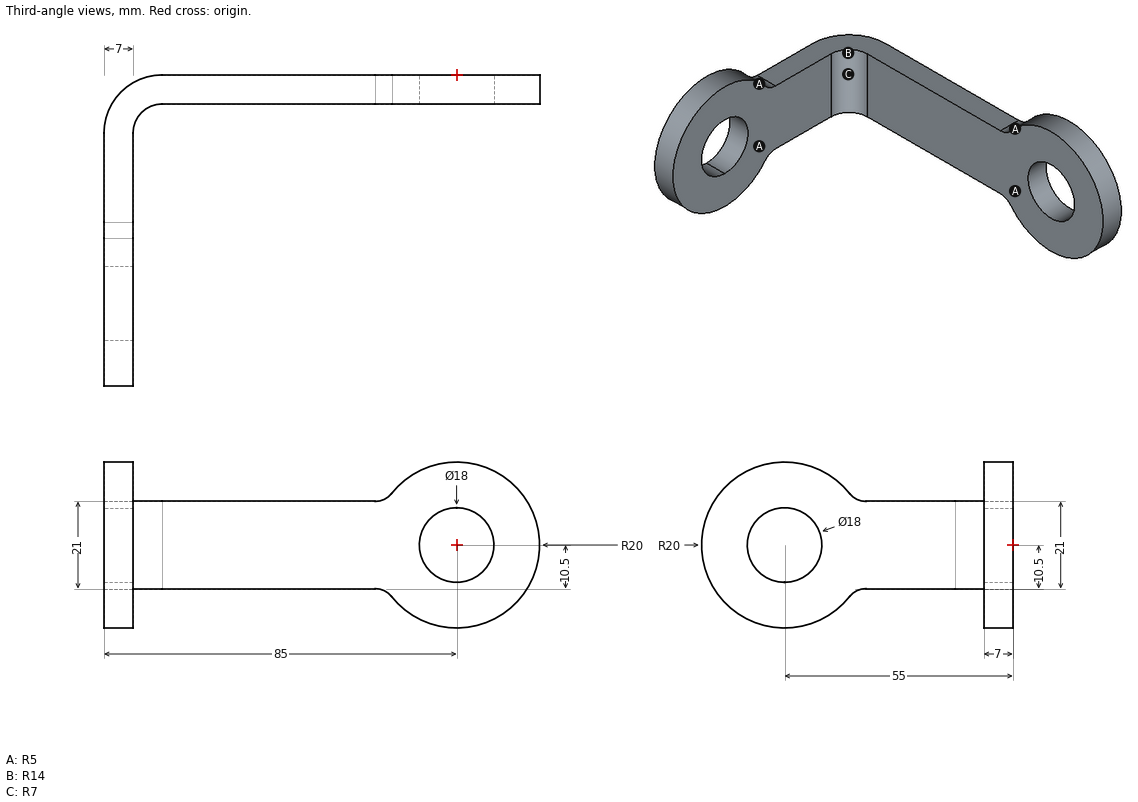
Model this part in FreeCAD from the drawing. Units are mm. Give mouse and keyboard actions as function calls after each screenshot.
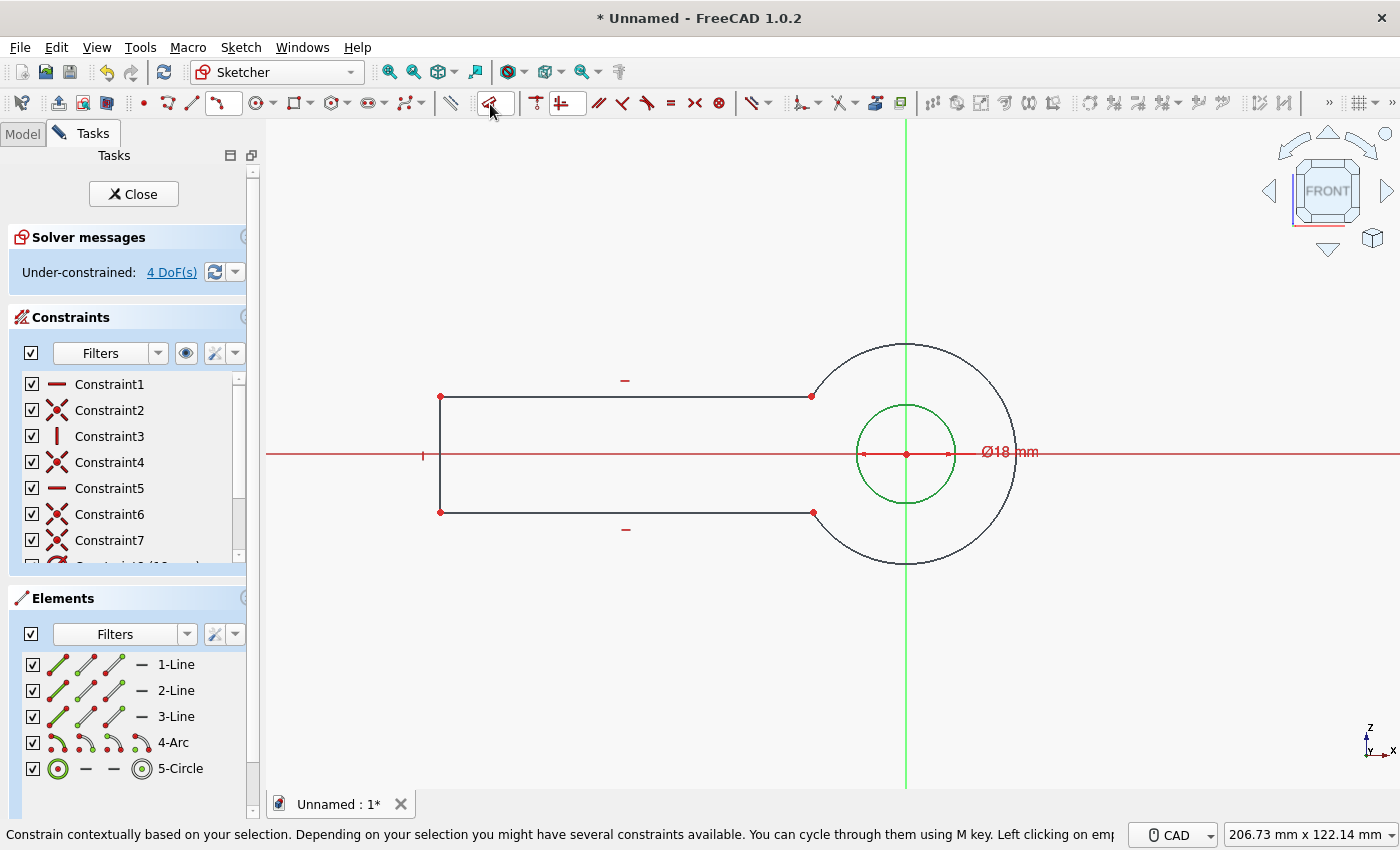
click(963, 548)
click(980, 575)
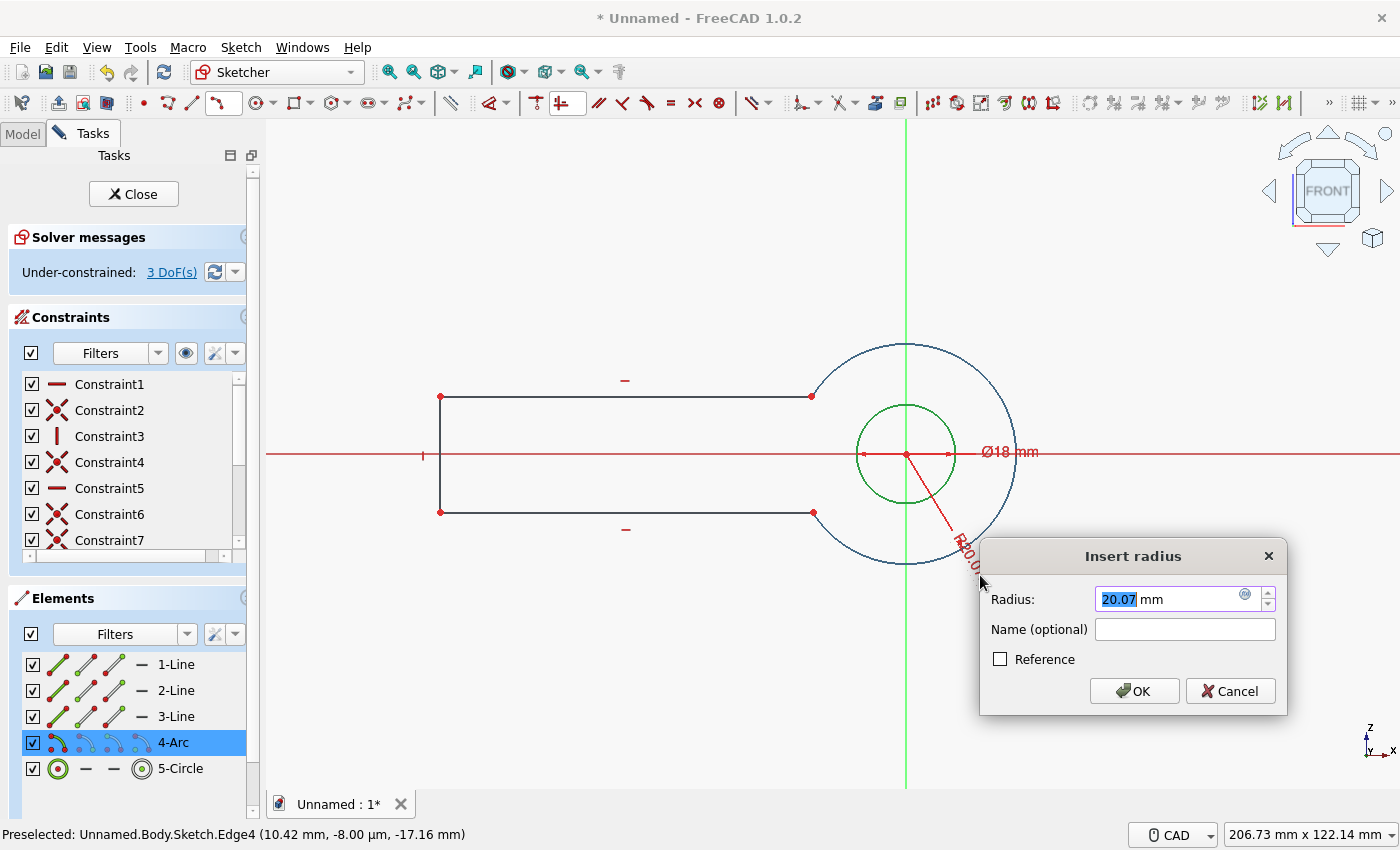
text(20)
key(Return)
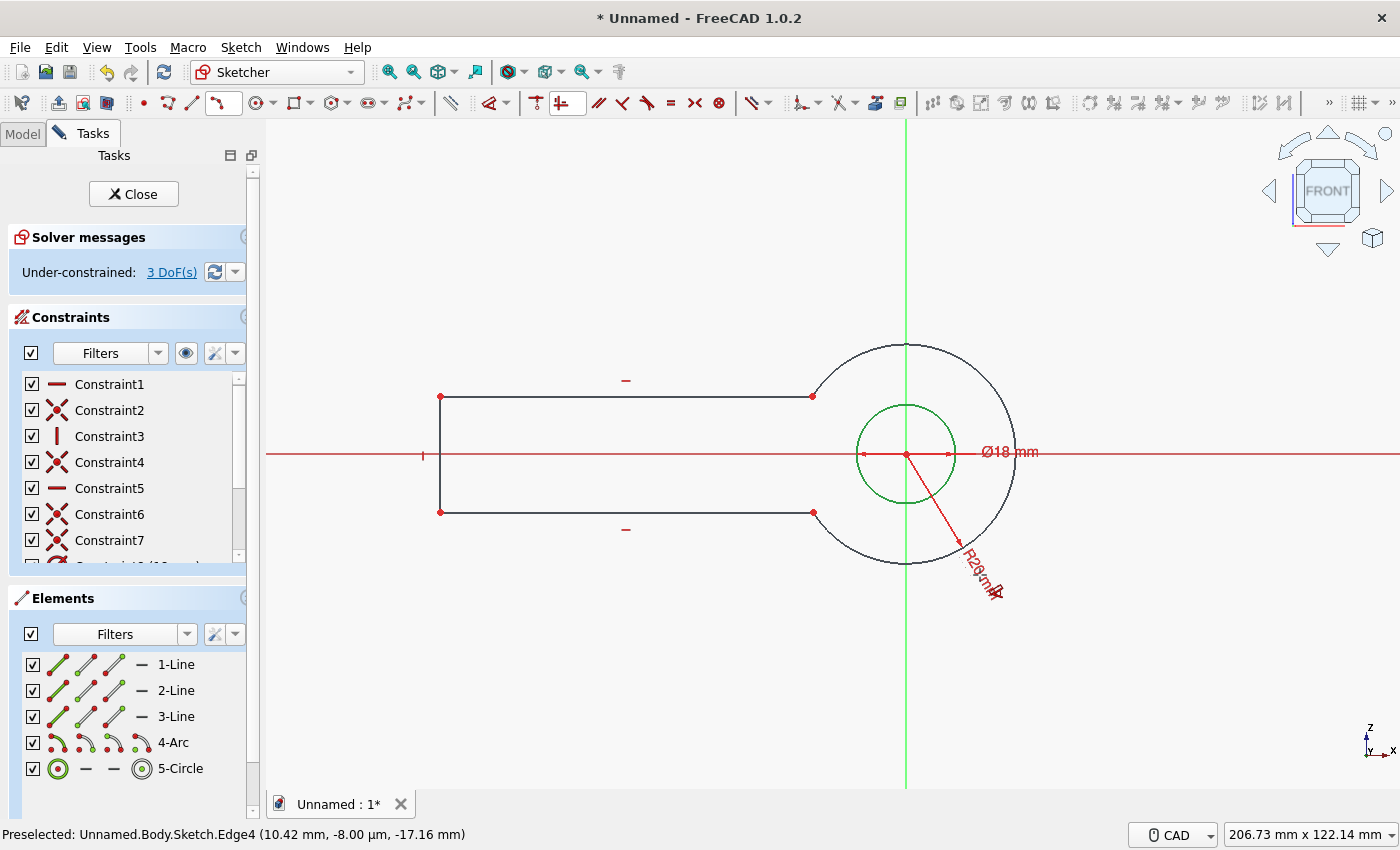
click(440, 478)
click(406, 428)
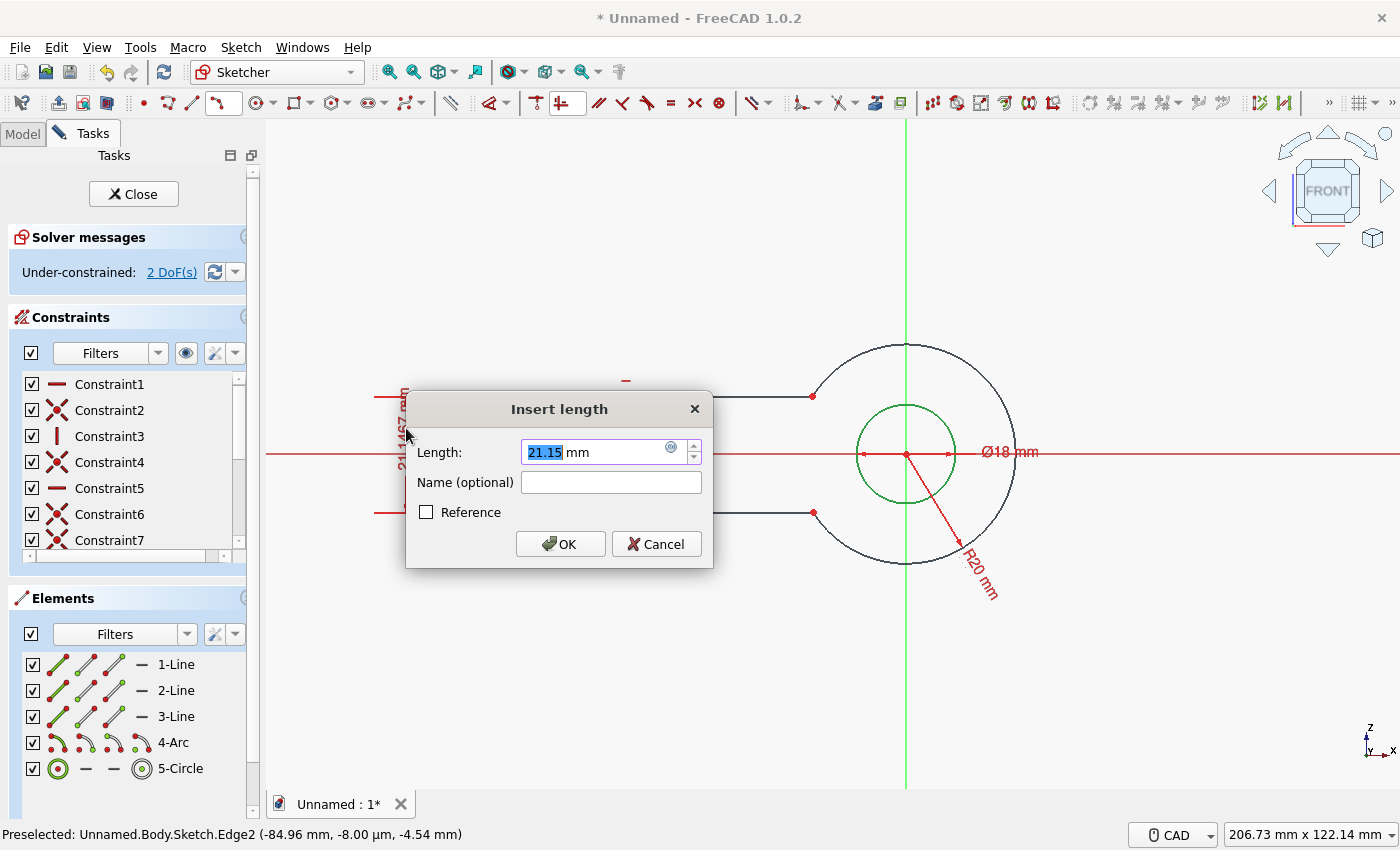
text(21)
key(Return)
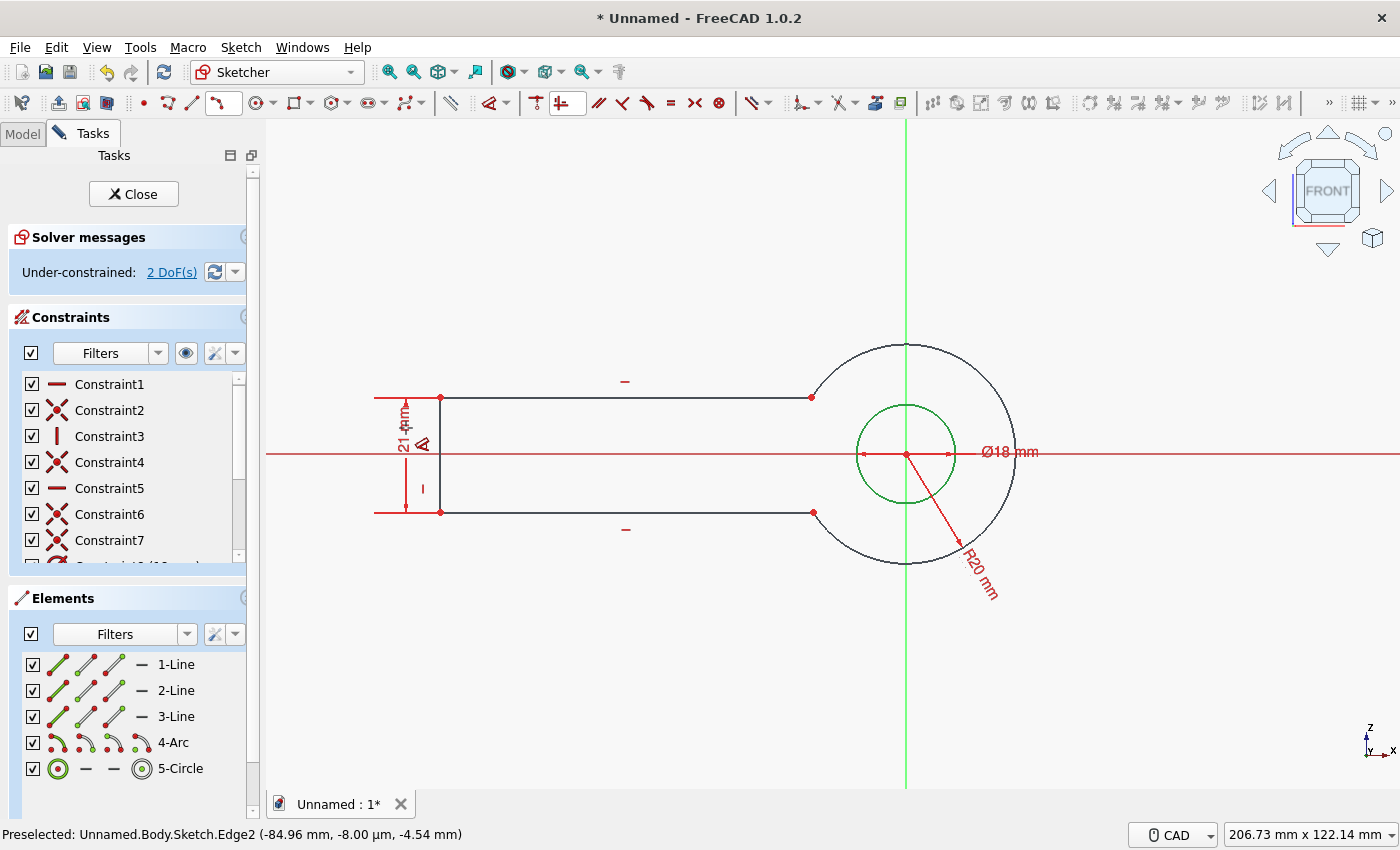
click(440, 513)
click(673, 547)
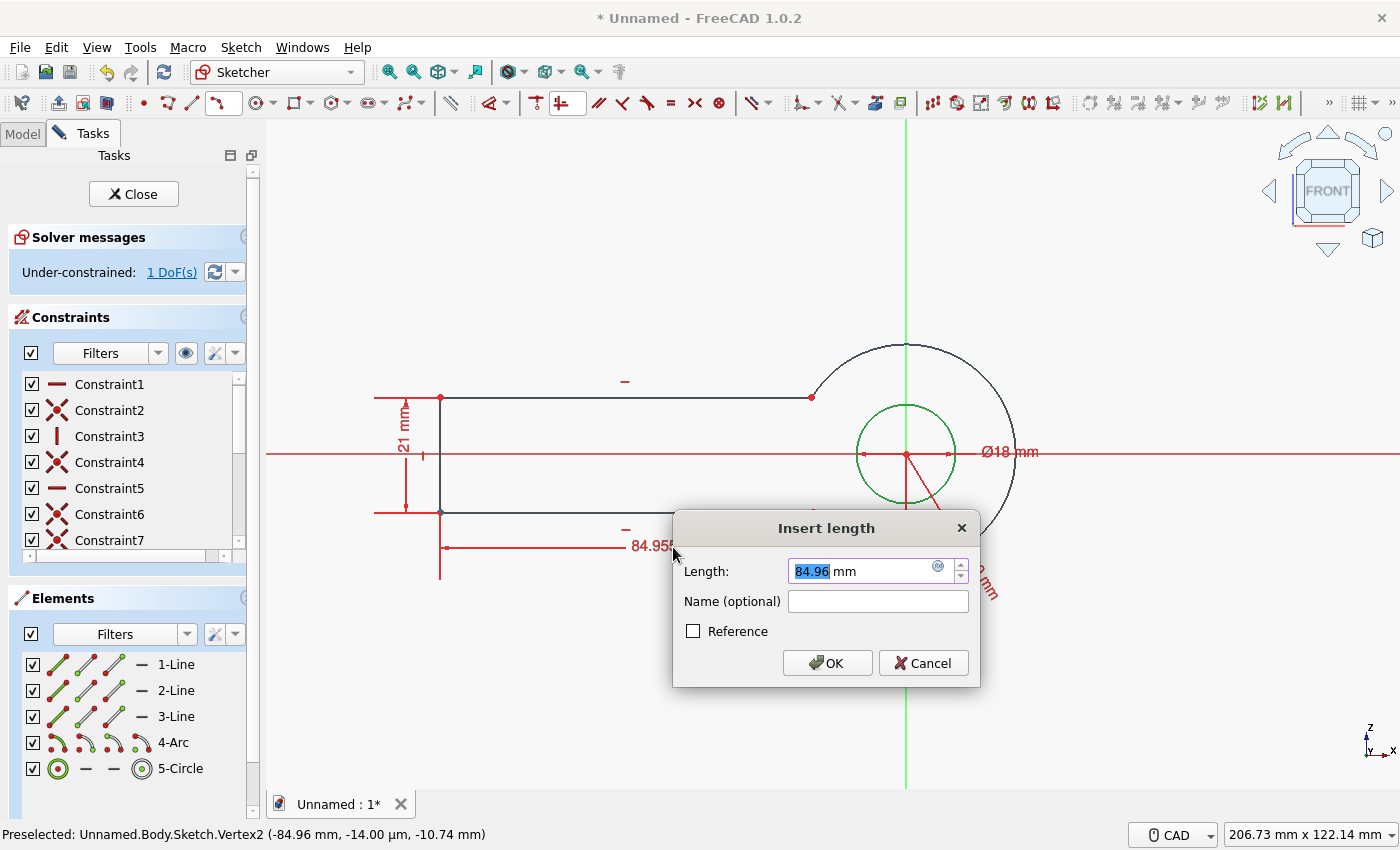
text(85)
key(Return)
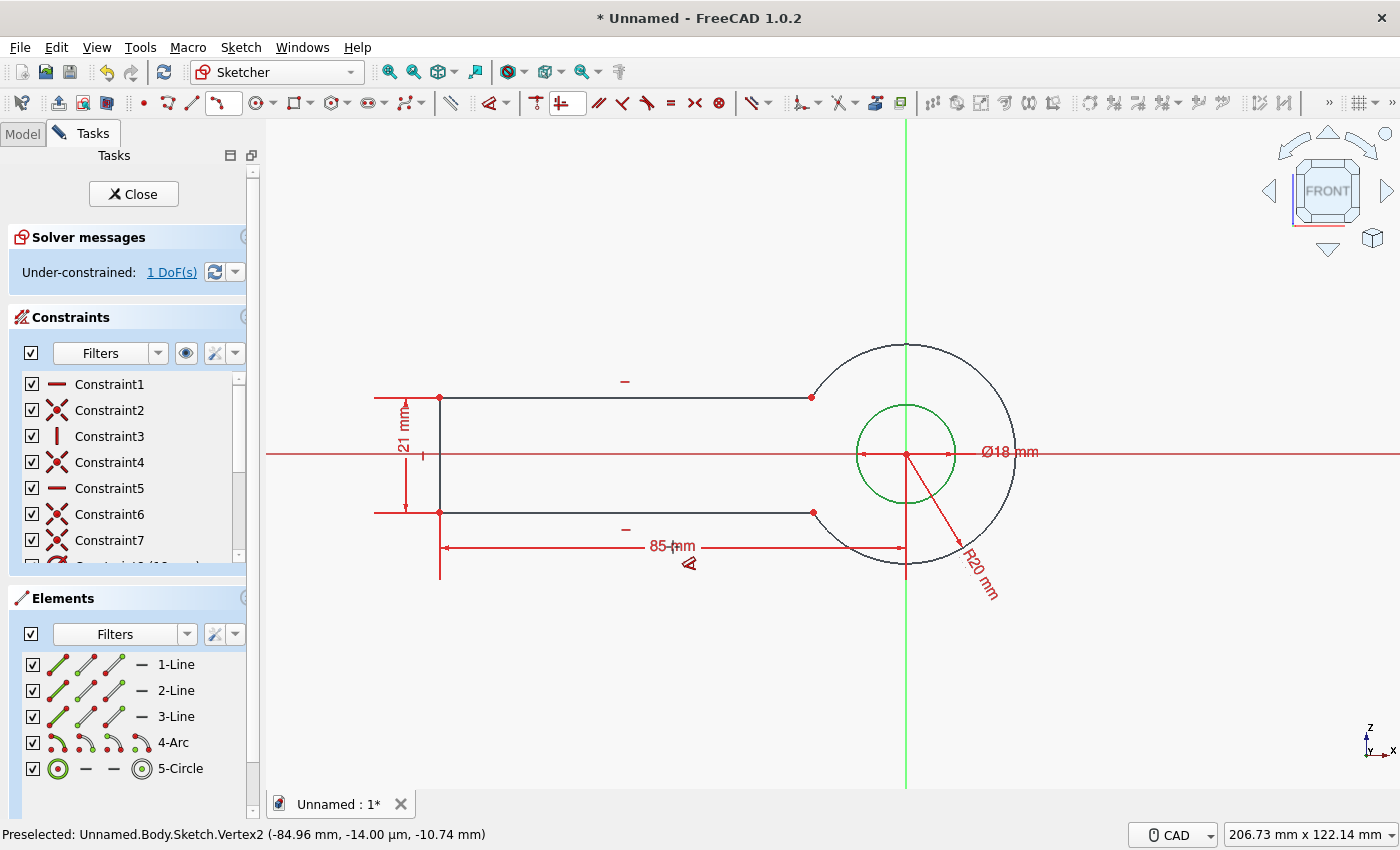
click(813, 513)
click(779, 484)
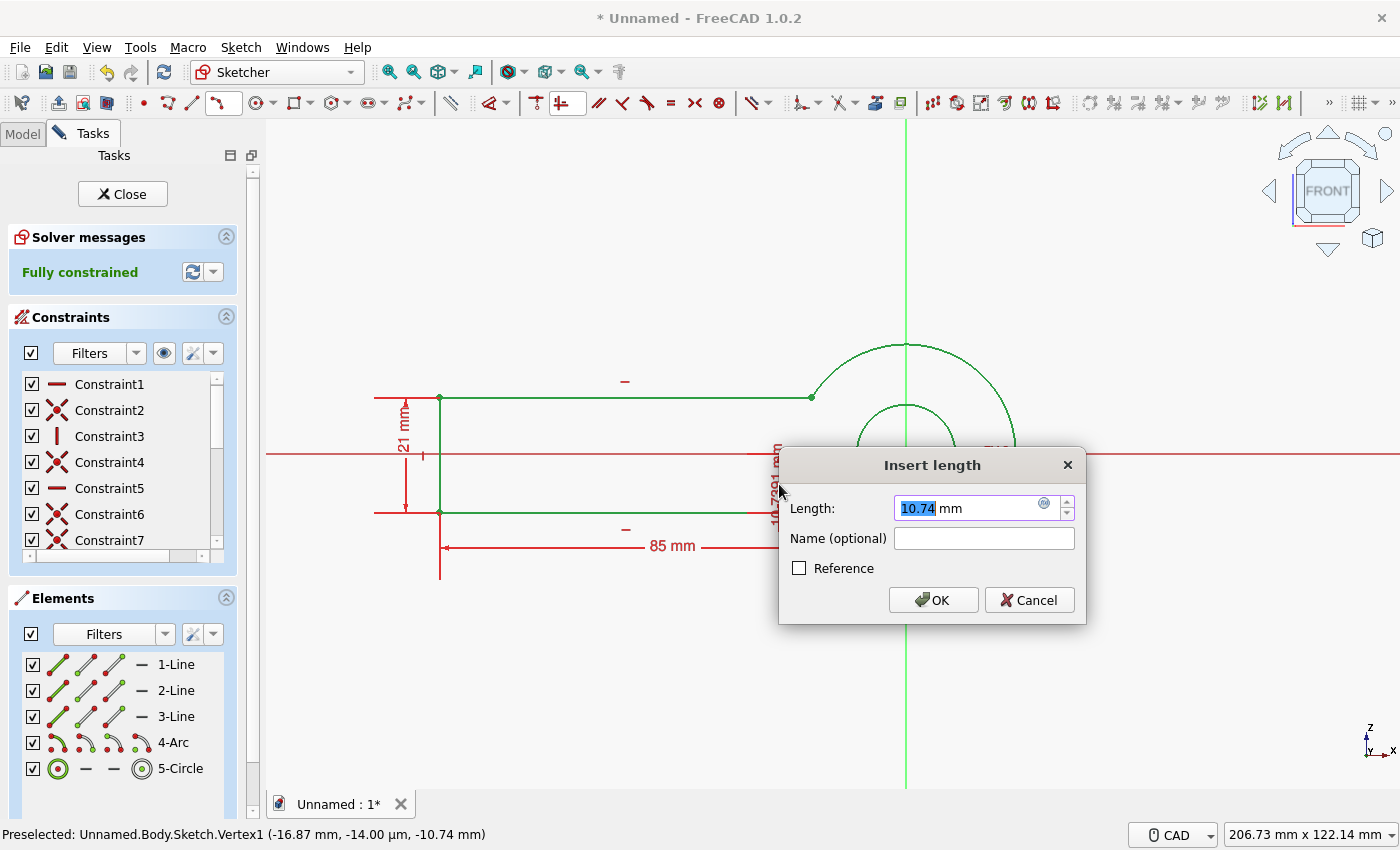
text(10.5)
key(Return)
key(Escape)